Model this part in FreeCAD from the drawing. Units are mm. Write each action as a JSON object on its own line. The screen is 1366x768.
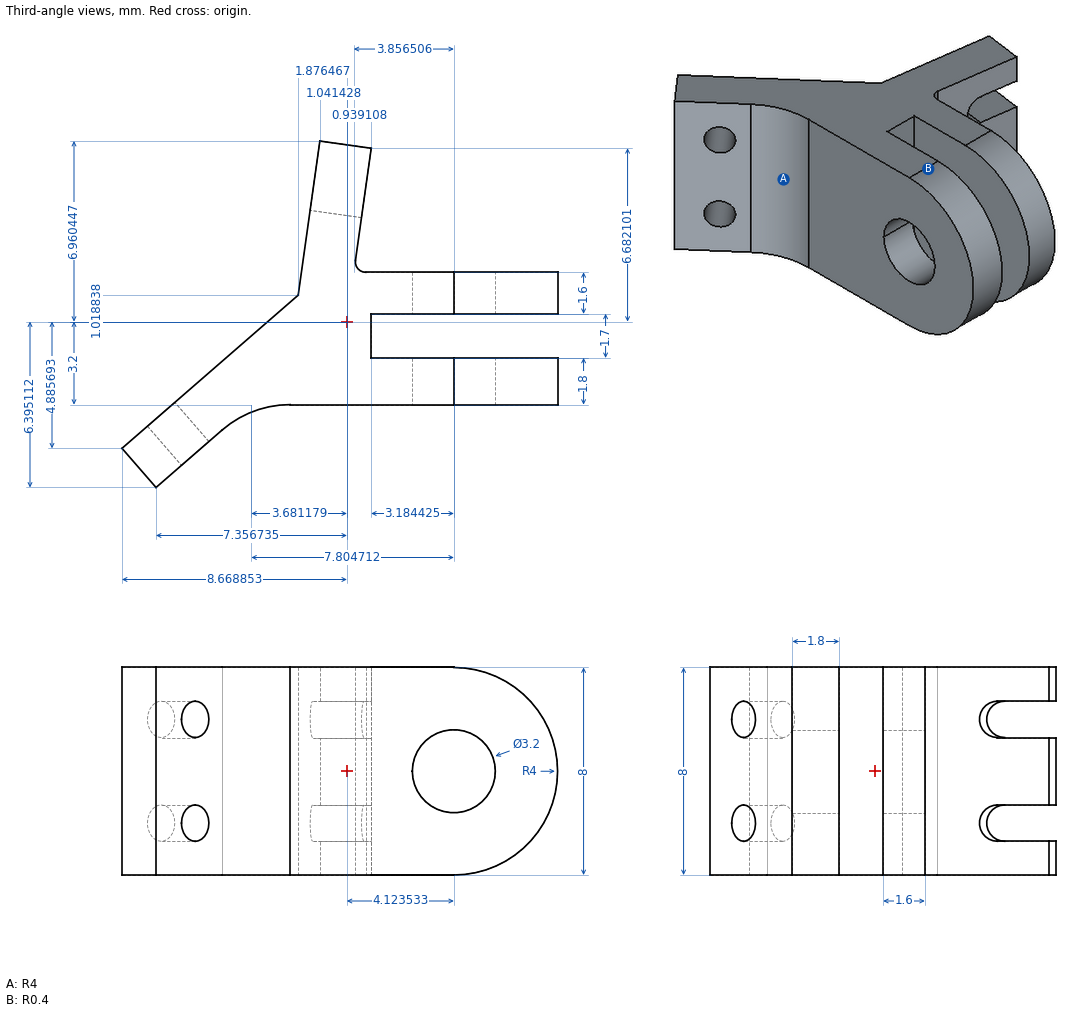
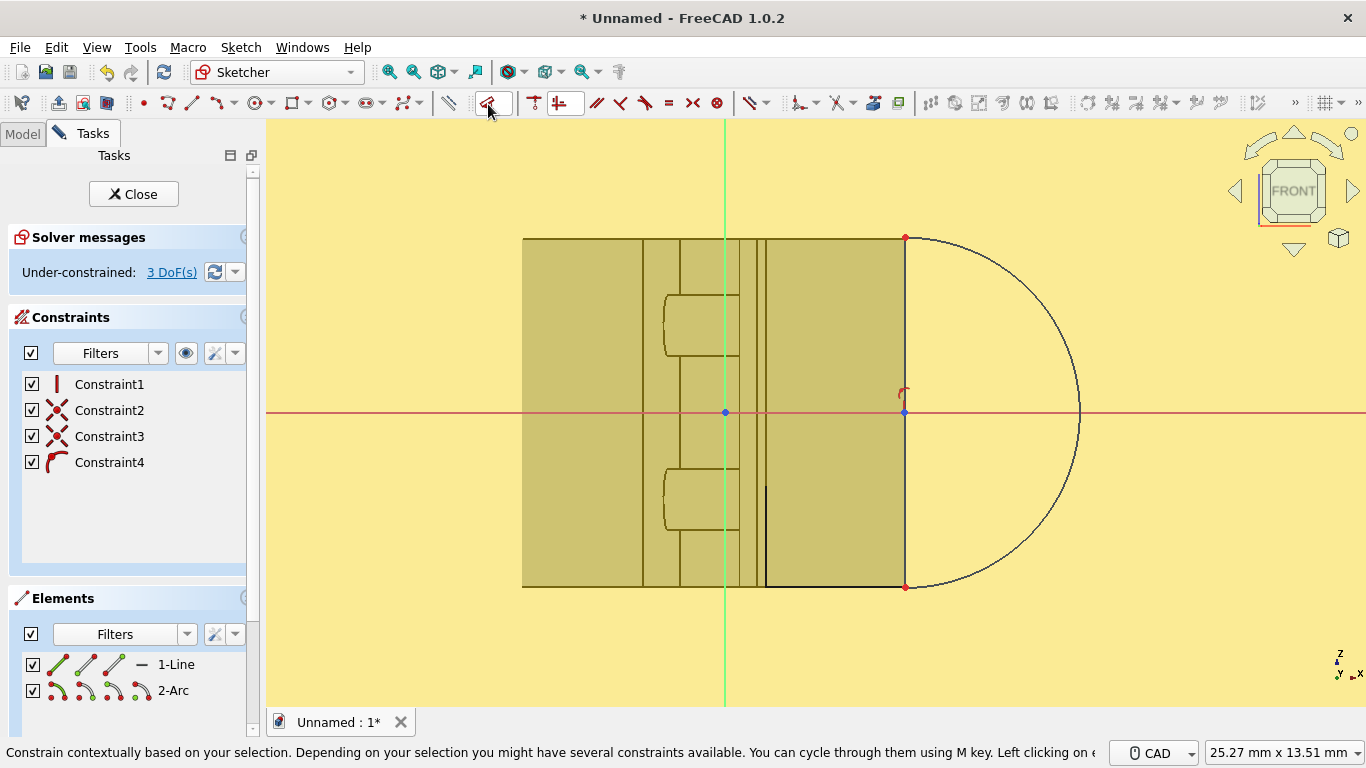
{"action": "left_click", "coordinate": [1046, 516]}
{"action": "left_click", "coordinate": [1072, 535]}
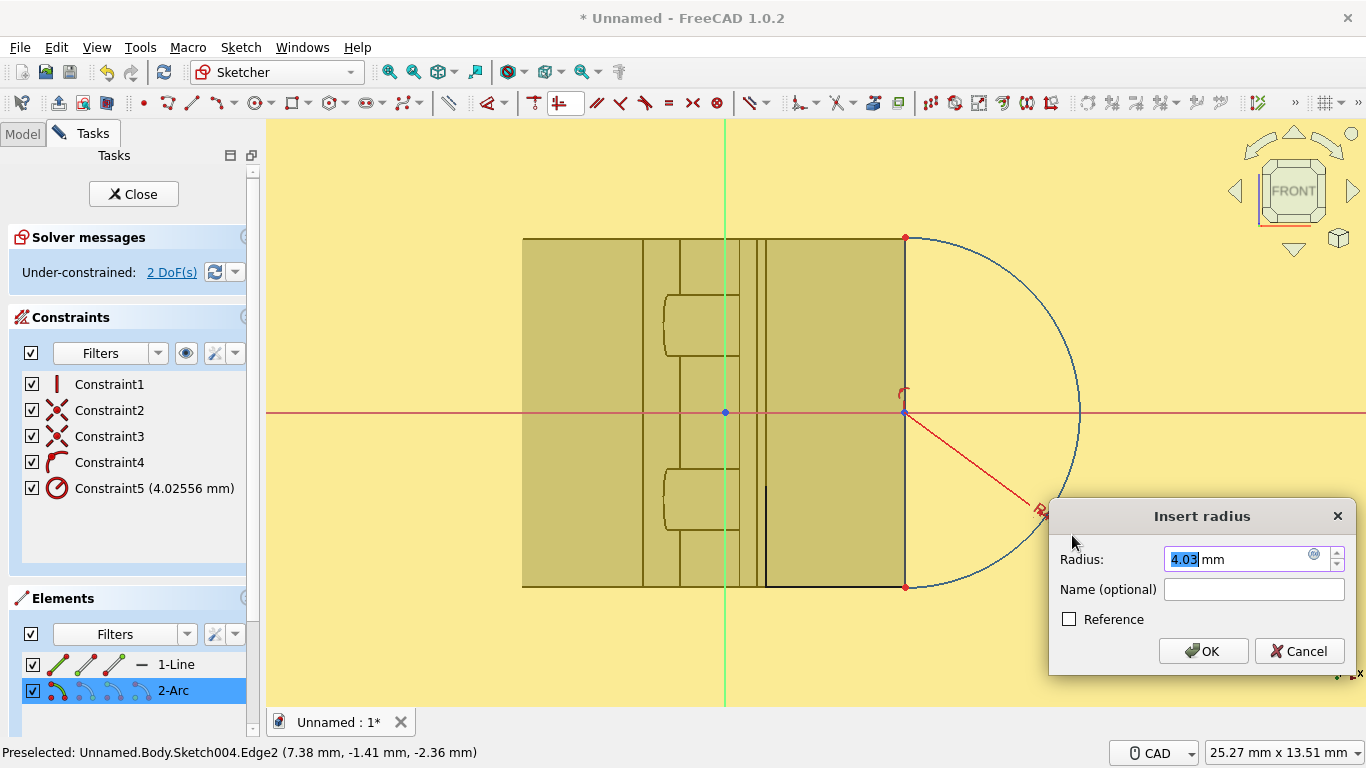
{"action": "type", "text": "4"}
{"action": "key", "text": "Return"}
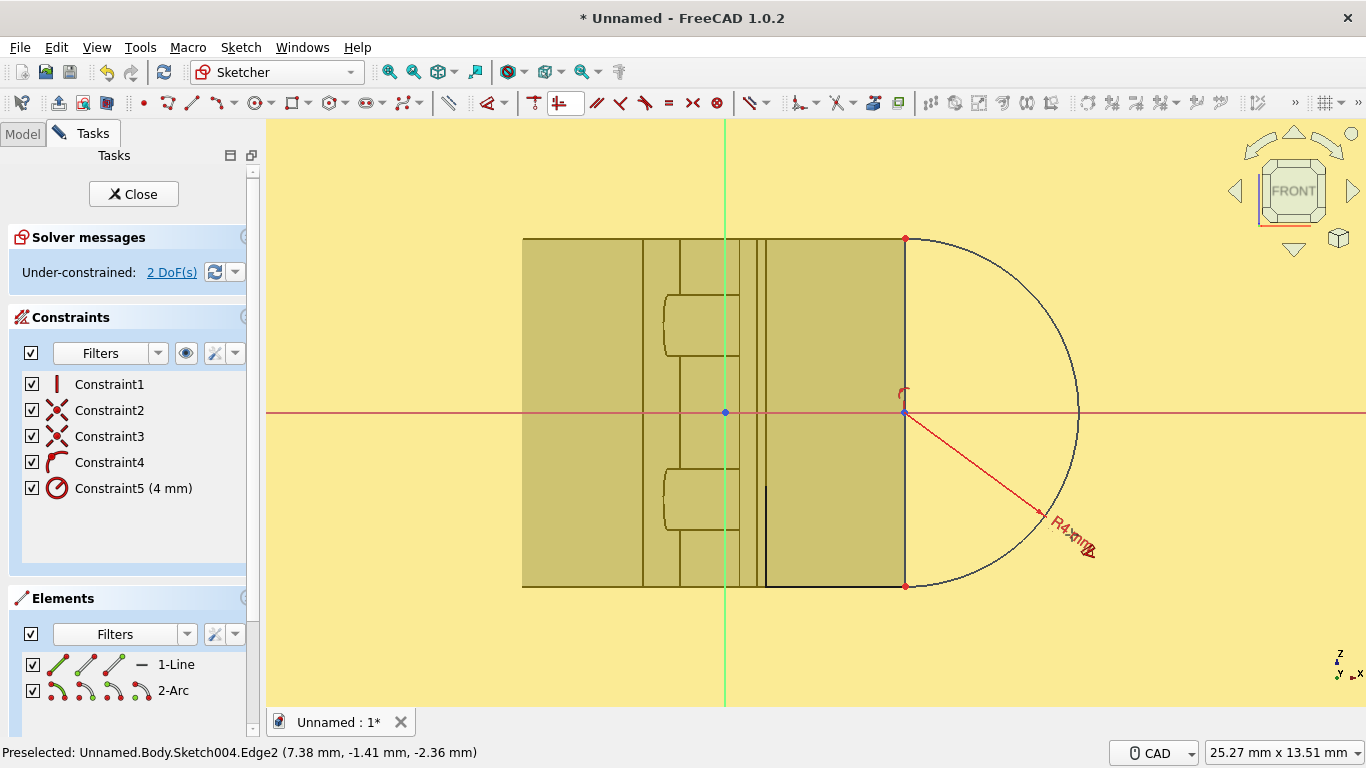
{"action": "left_click", "coordinate": [905, 587]}
{"action": "left_click", "coordinate": [815, 621]}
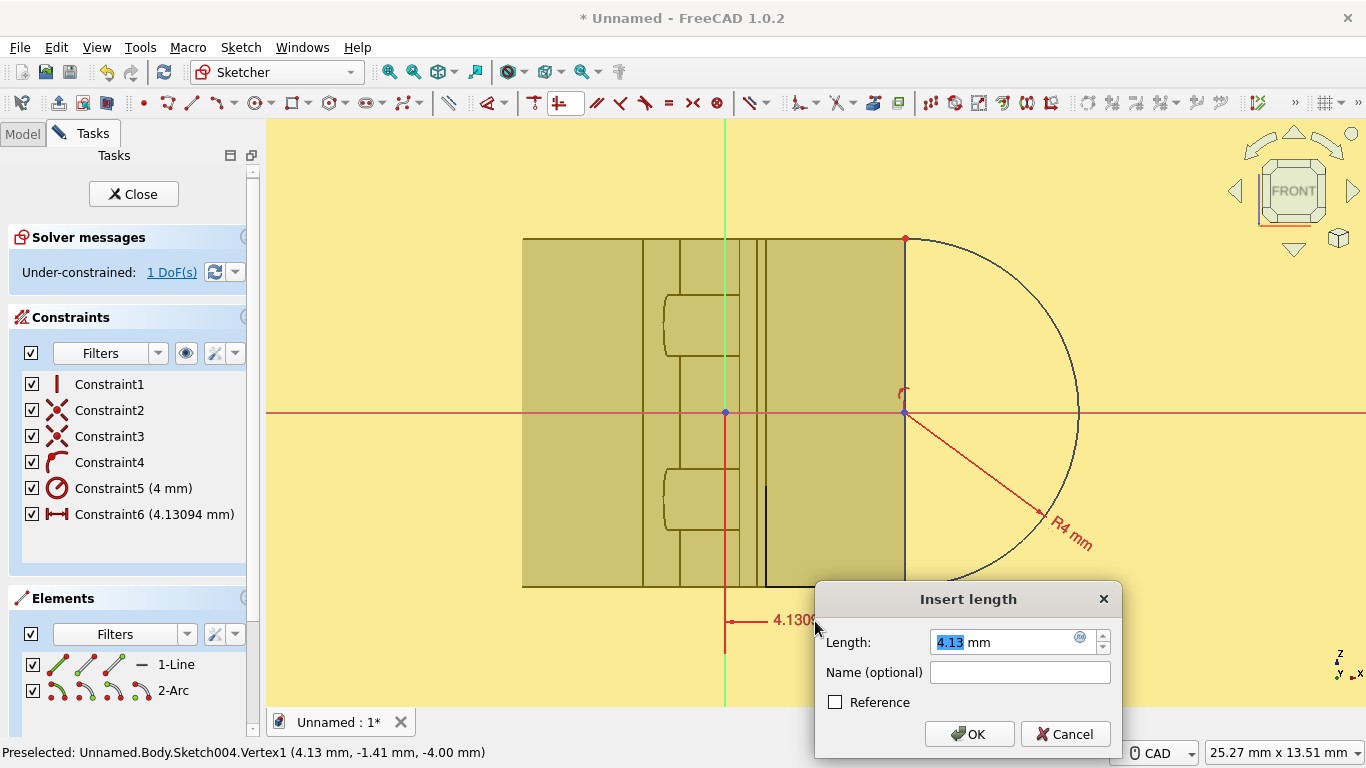
{"action": "type", "text": "4.123533"}
{"action": "key", "text": "Return"}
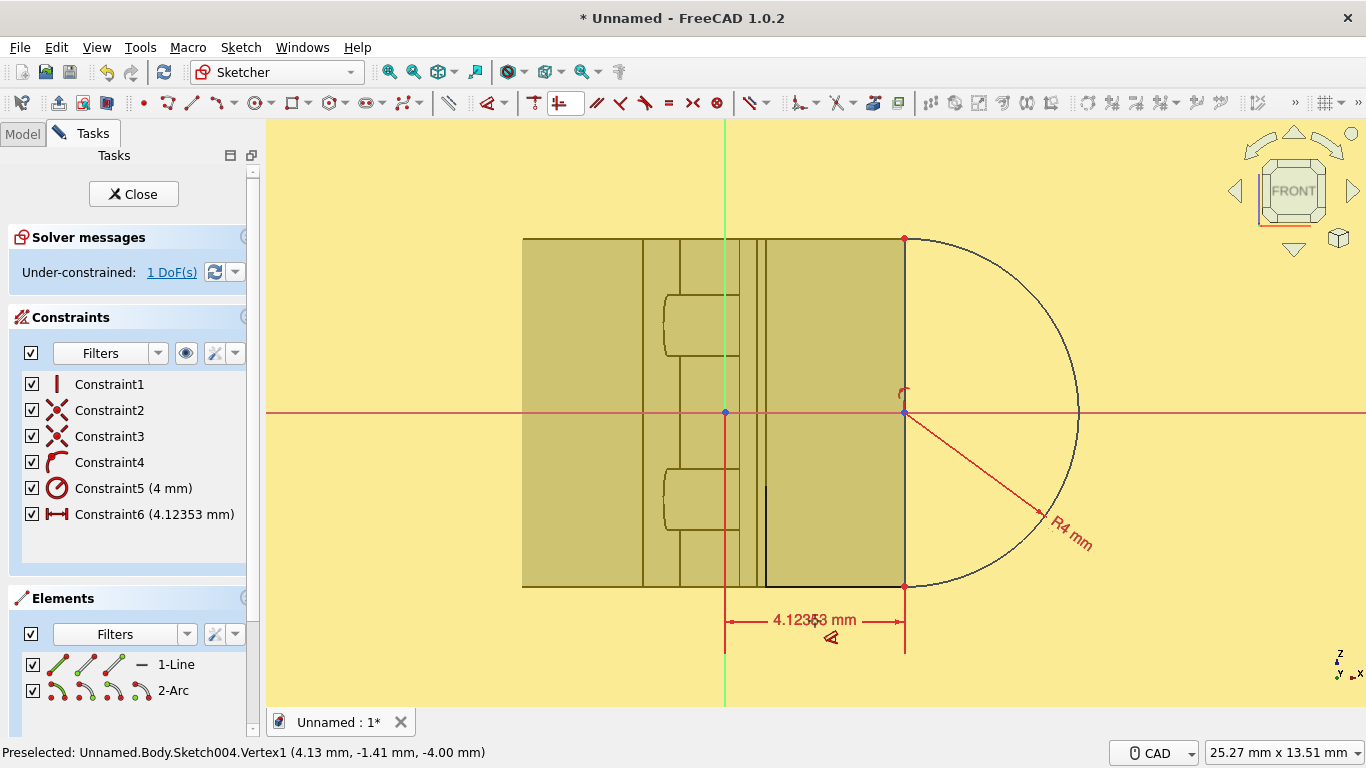
{"action": "left_click", "coordinate": [905, 413]}
{"action": "left_click", "coordinate": [815, 447]}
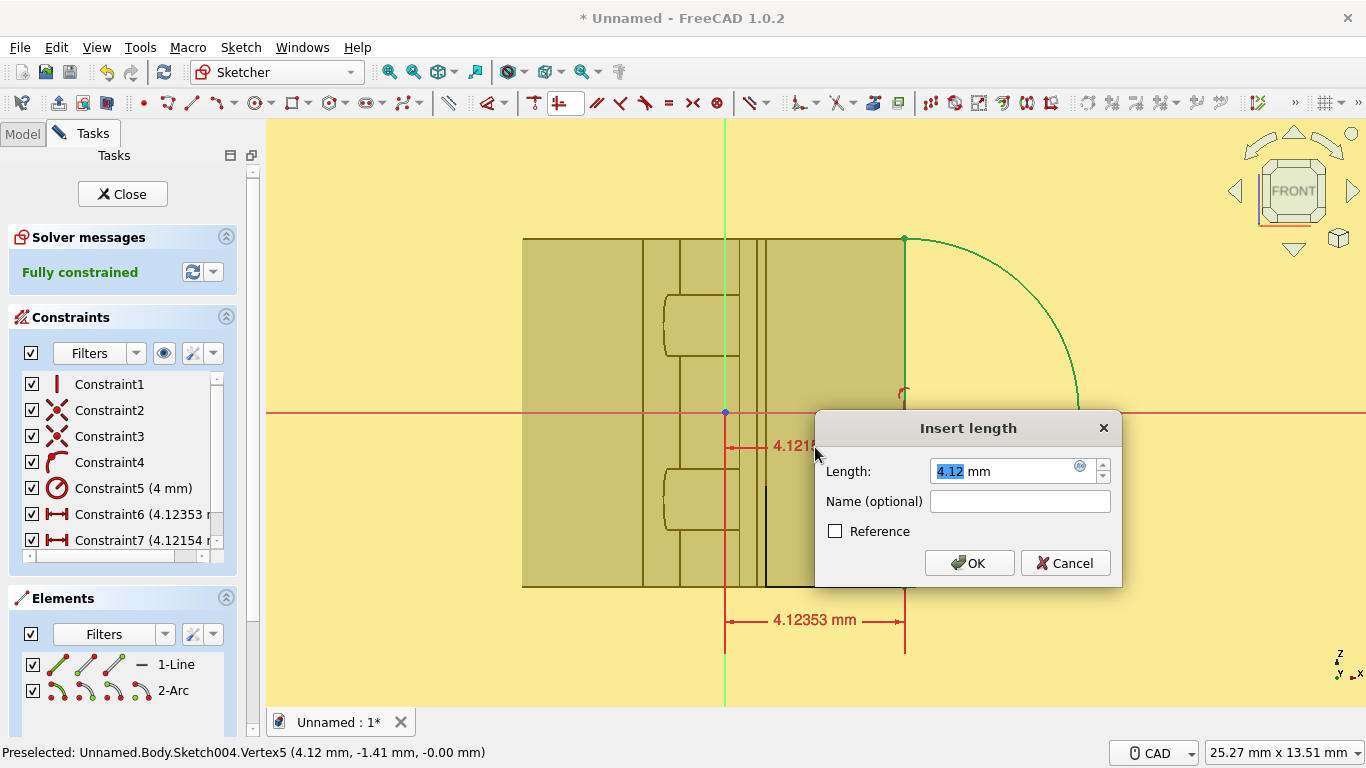
{"action": "type", "text": "4.123533"}
{"action": "key", "text": "Return"}
{"action": "key", "text": "Escape"}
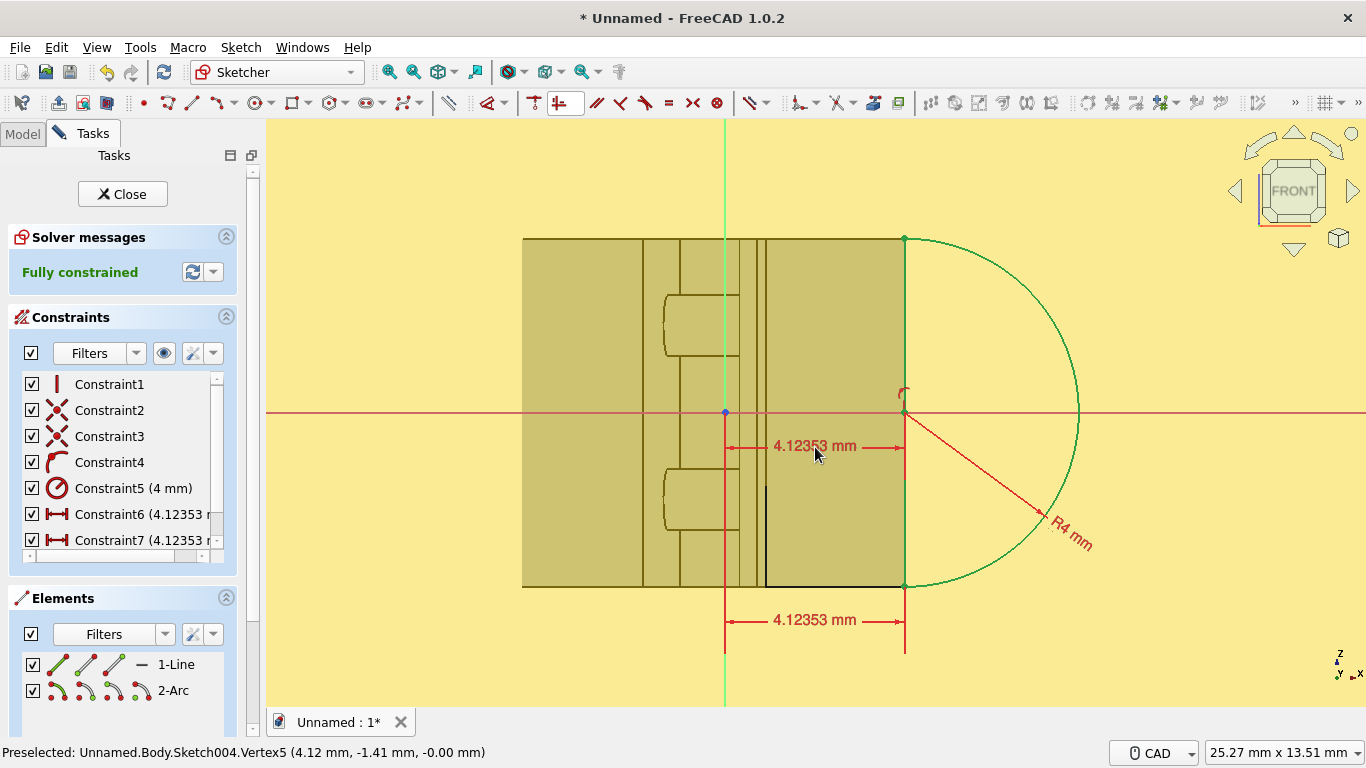
{"action": "left_click", "coordinate": [123, 194]}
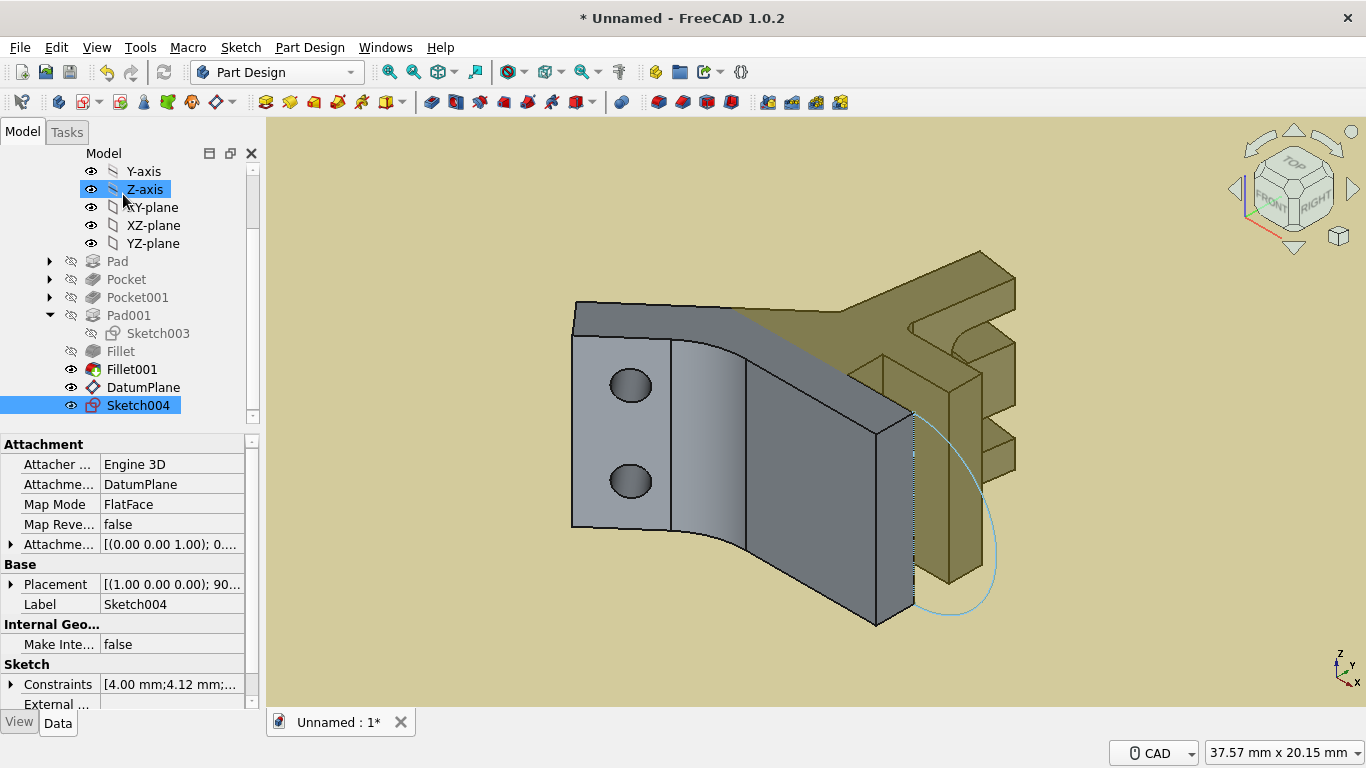
{"action": "left_click", "coordinate": [266, 102]}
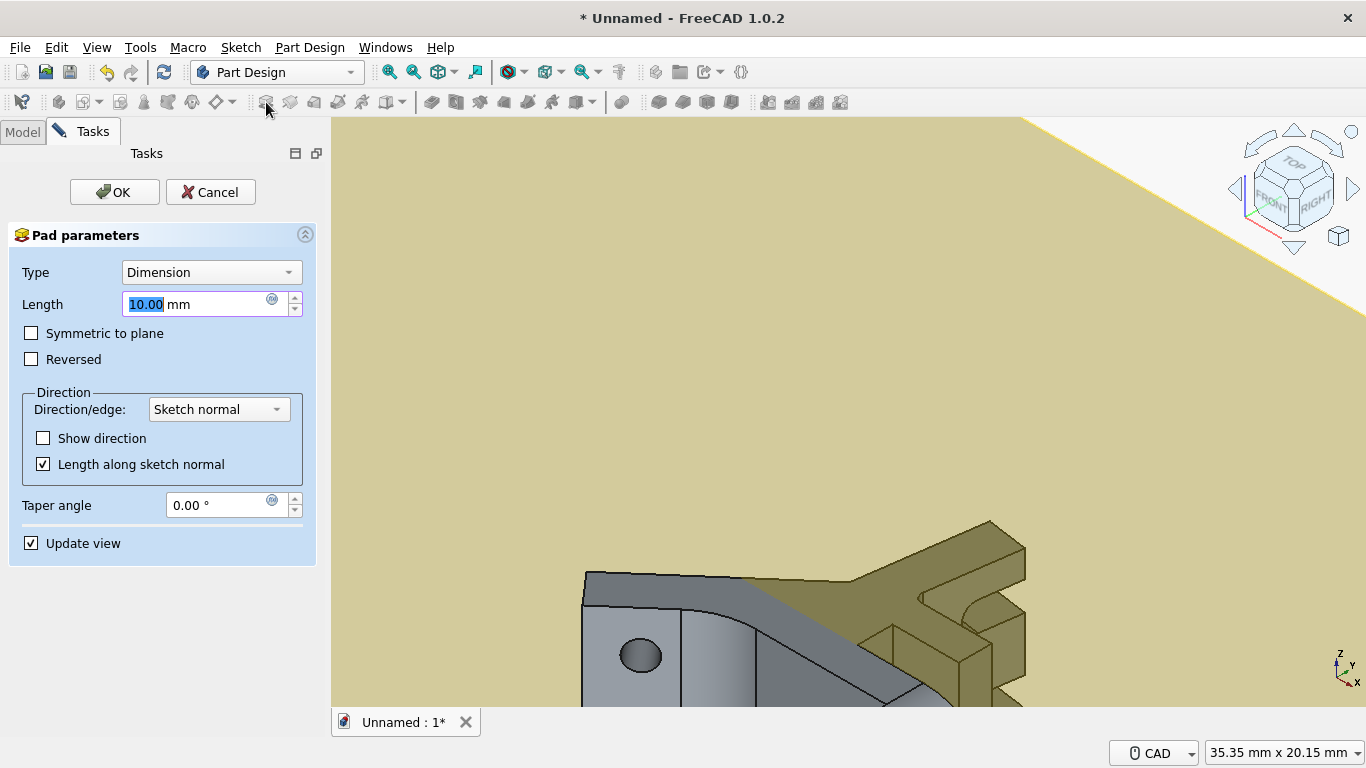
{"action": "type", "text": "1.8"}
{"action": "key", "text": "Tab"}